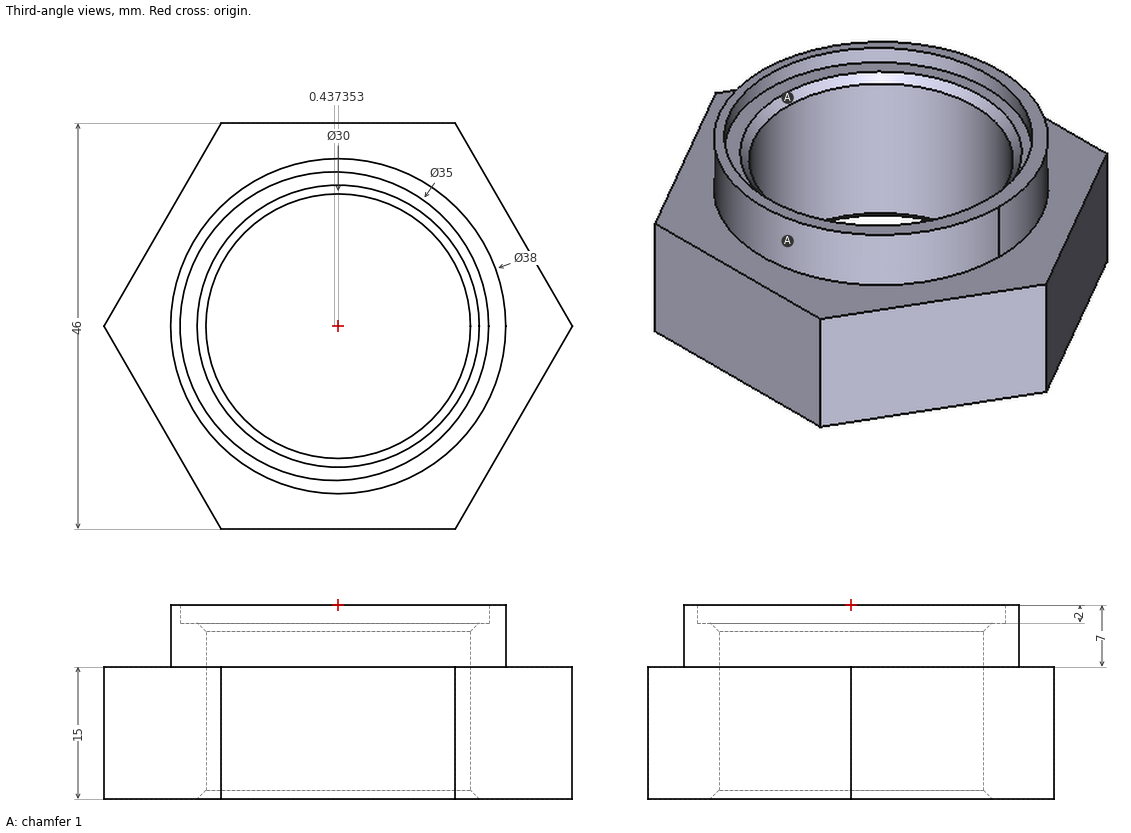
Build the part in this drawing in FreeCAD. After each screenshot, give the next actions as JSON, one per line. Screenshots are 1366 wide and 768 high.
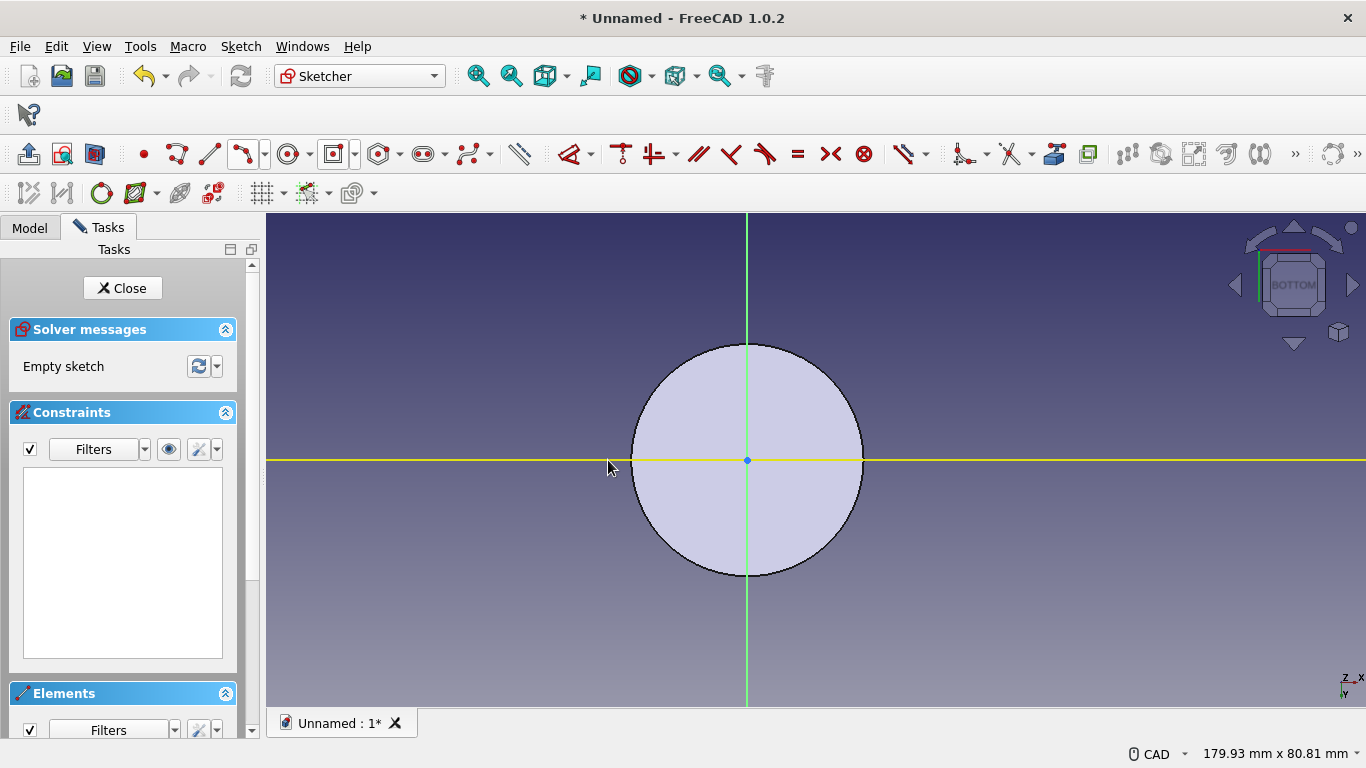
{"action": "left_click", "coordinate": [378, 154]}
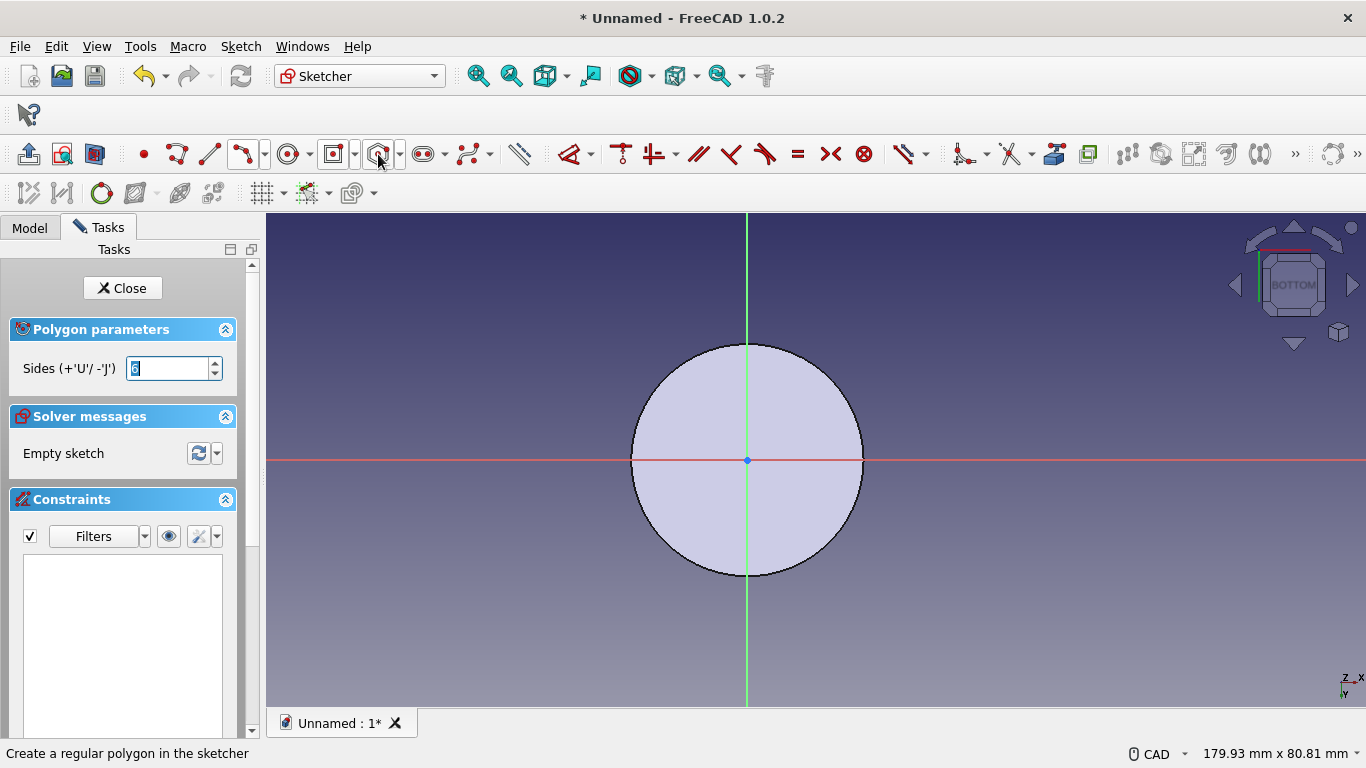
{"action": "left_click", "coordinate": [747, 460]}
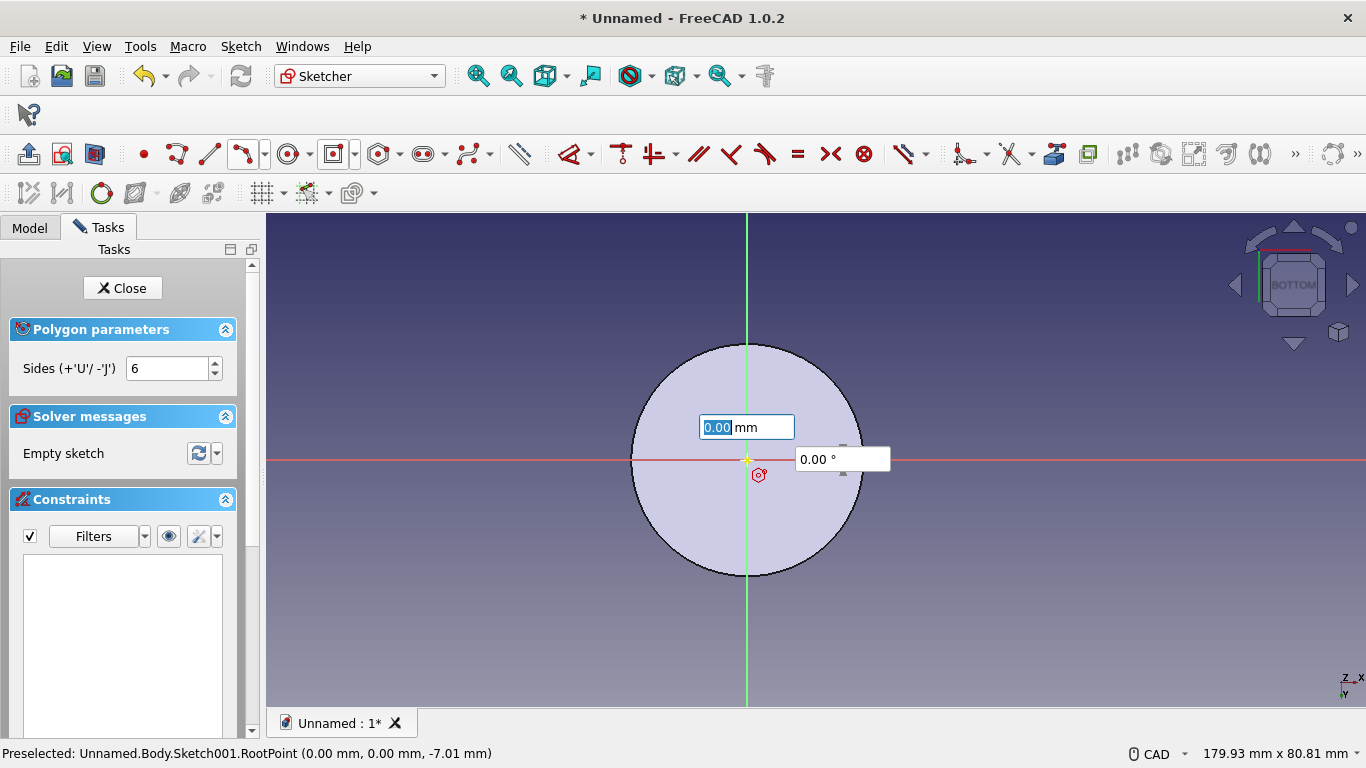
{"action": "left_click", "coordinate": [585, 460]}
{"action": "right_click", "coordinate": [585, 460]}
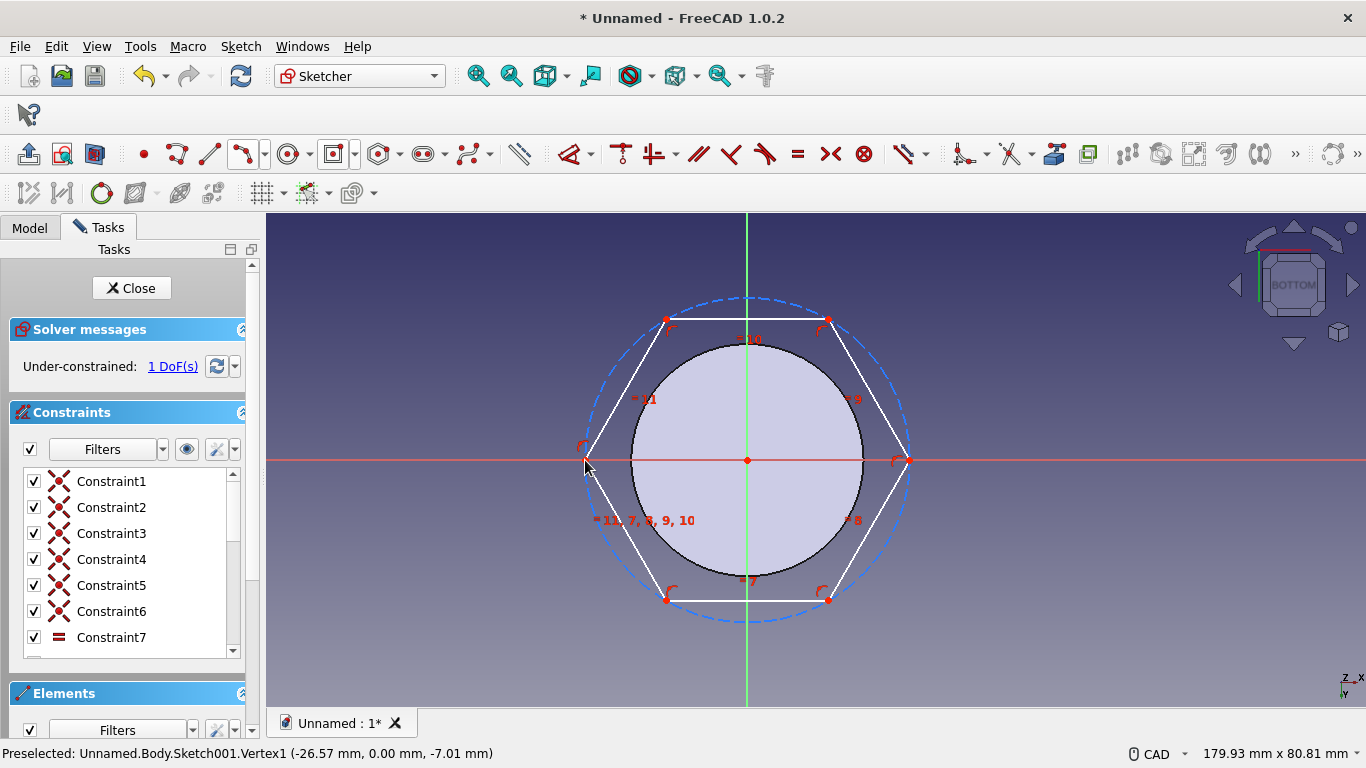
{"action": "left_click", "coordinate": [568, 154]}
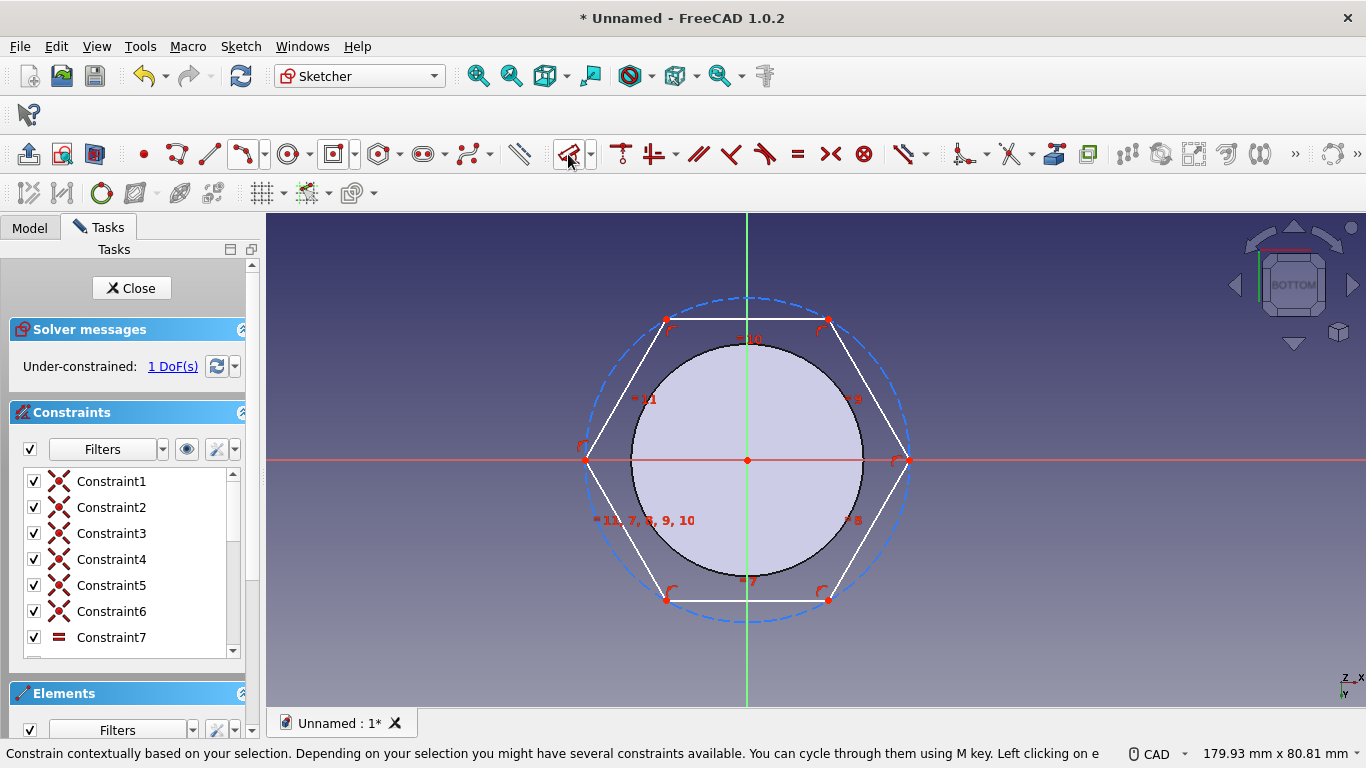
{"action": "left_click", "coordinate": [666, 601]}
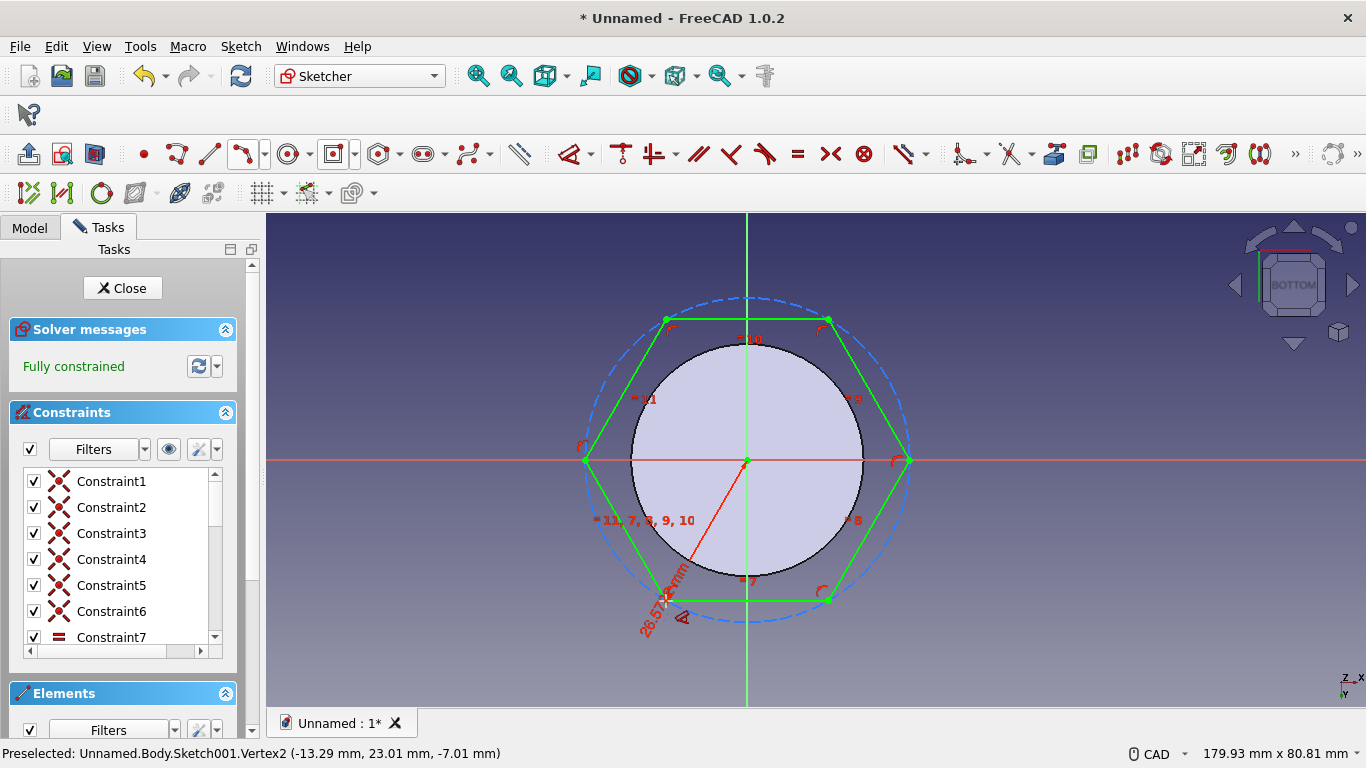
{"action": "left_click", "coordinate": [829, 319]}
{"action": "left_click", "coordinate": [911, 395]}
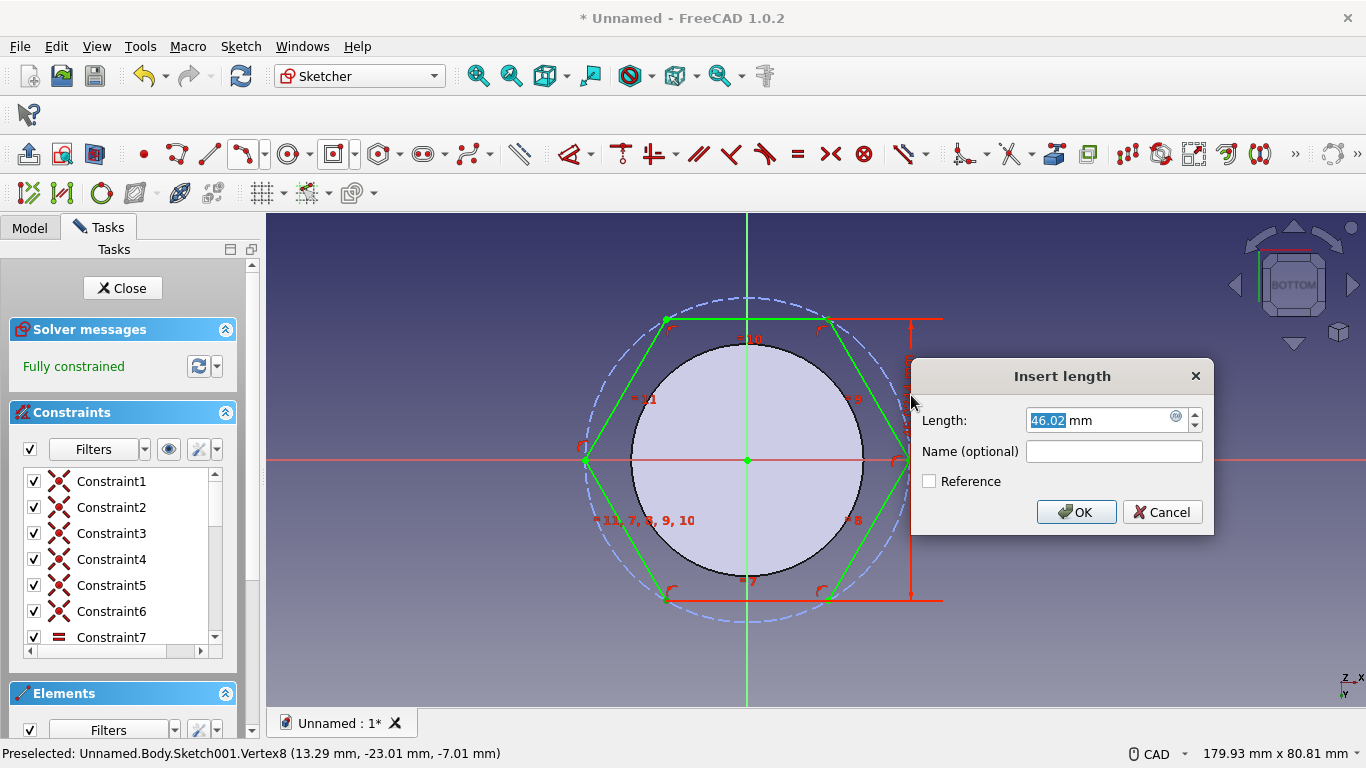
{"action": "type", "text": "46"}
{"action": "key", "text": "Return"}
{"action": "key", "text": "Escape"}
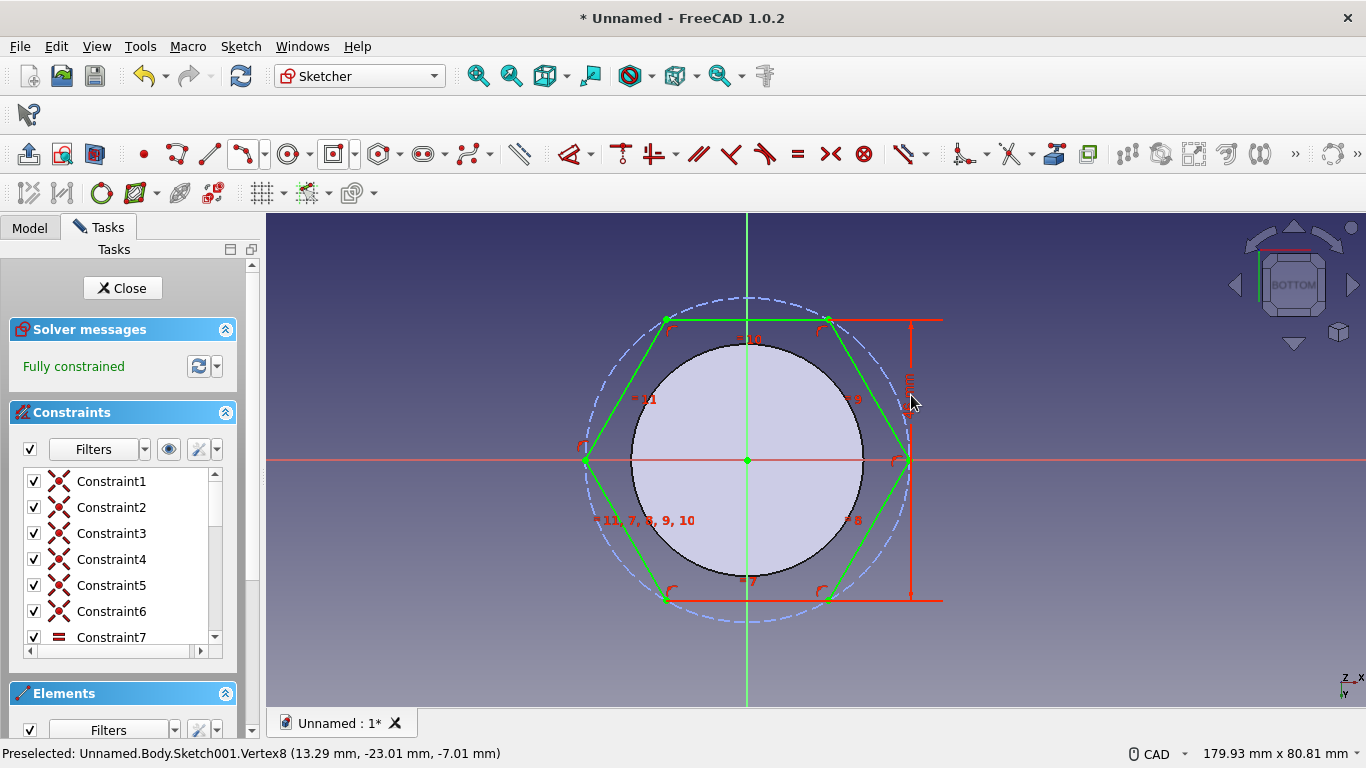
{"action": "left_click", "coordinate": [123, 288]}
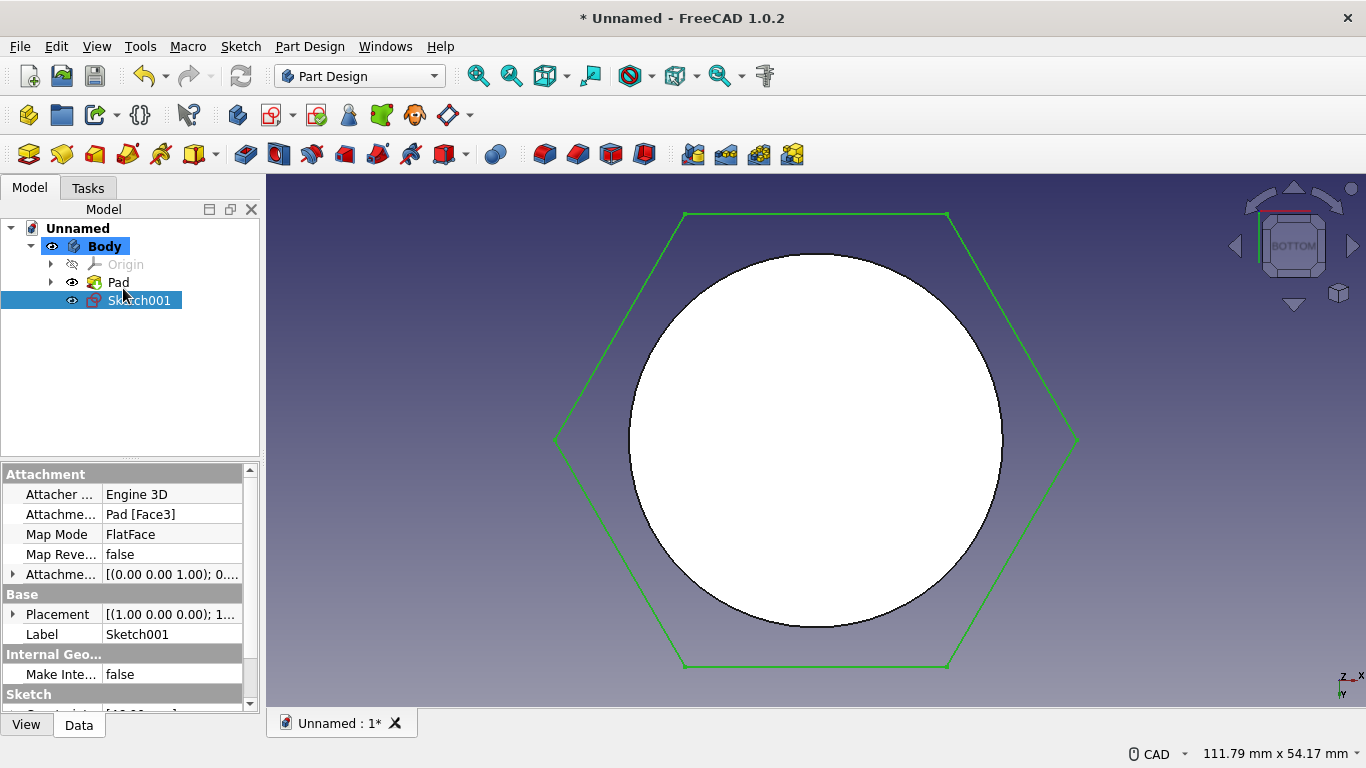
{"action": "left_click", "coordinate": [29, 154]}